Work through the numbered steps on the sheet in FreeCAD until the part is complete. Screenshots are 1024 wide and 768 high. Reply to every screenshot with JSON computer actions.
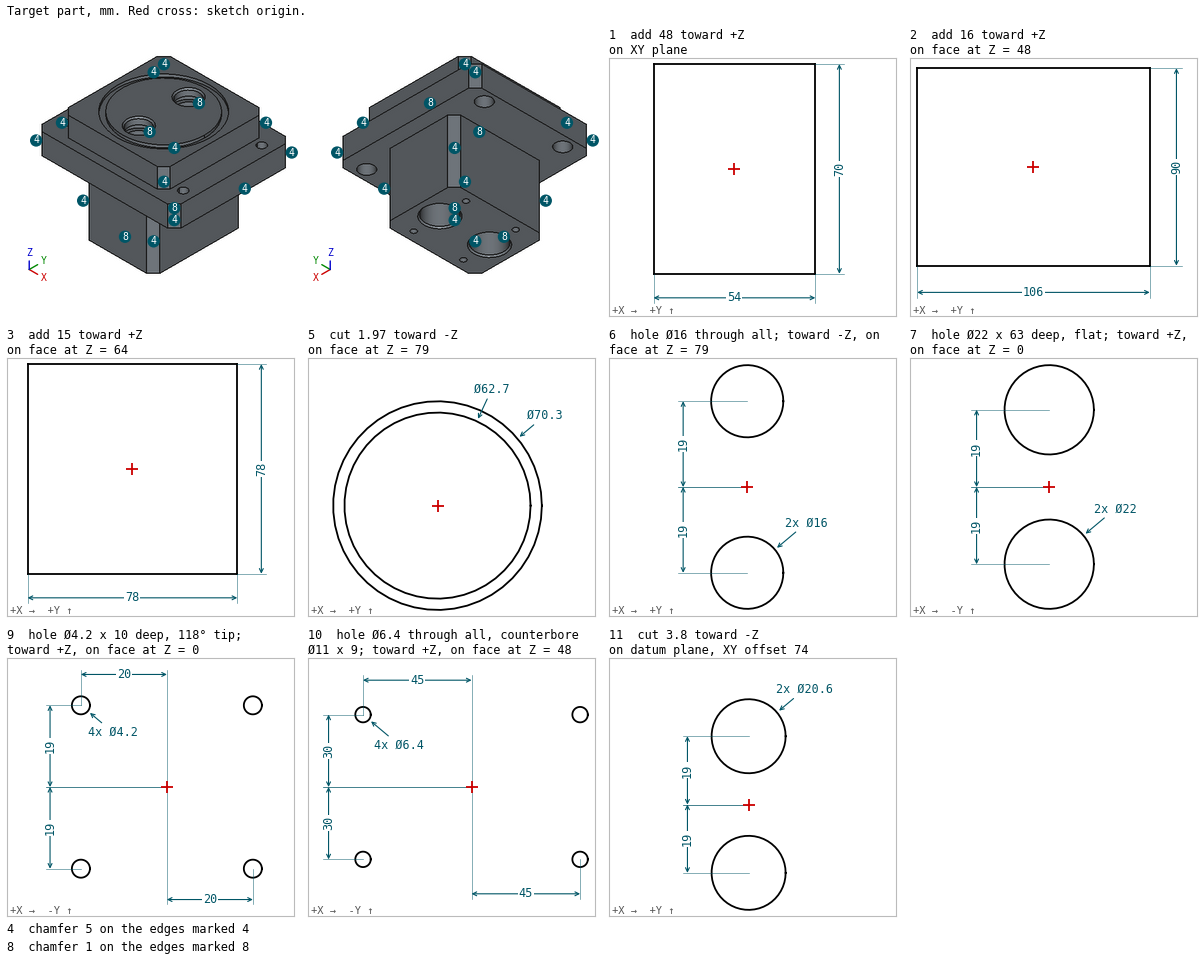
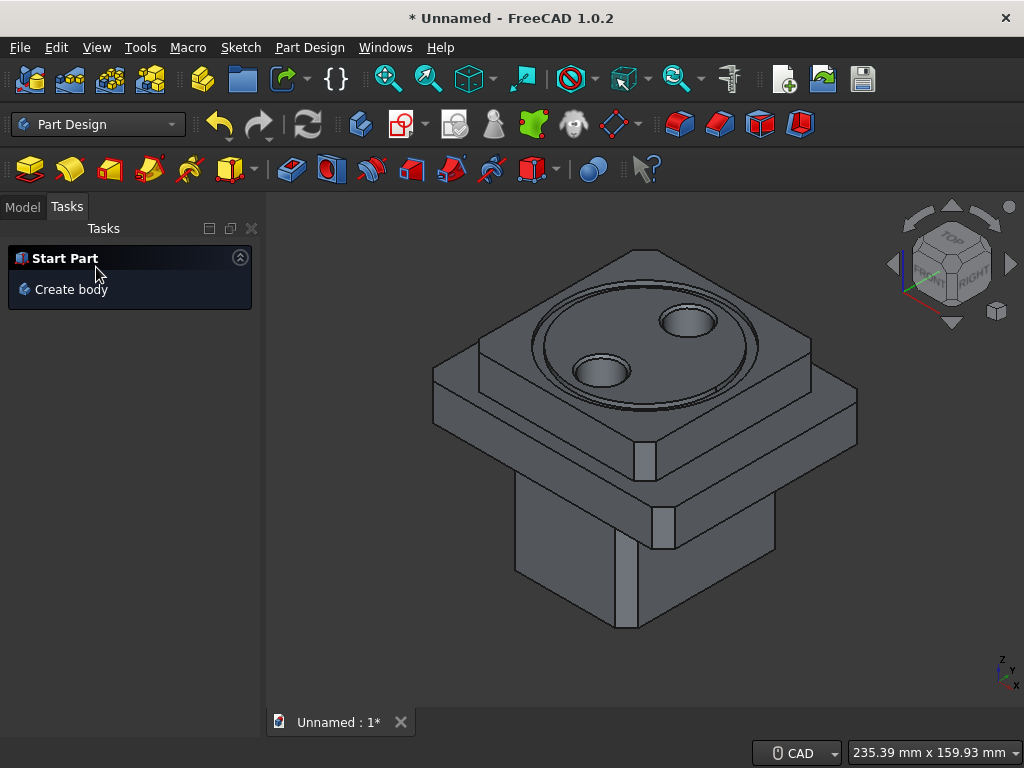
{"action": "key", "text": "5"}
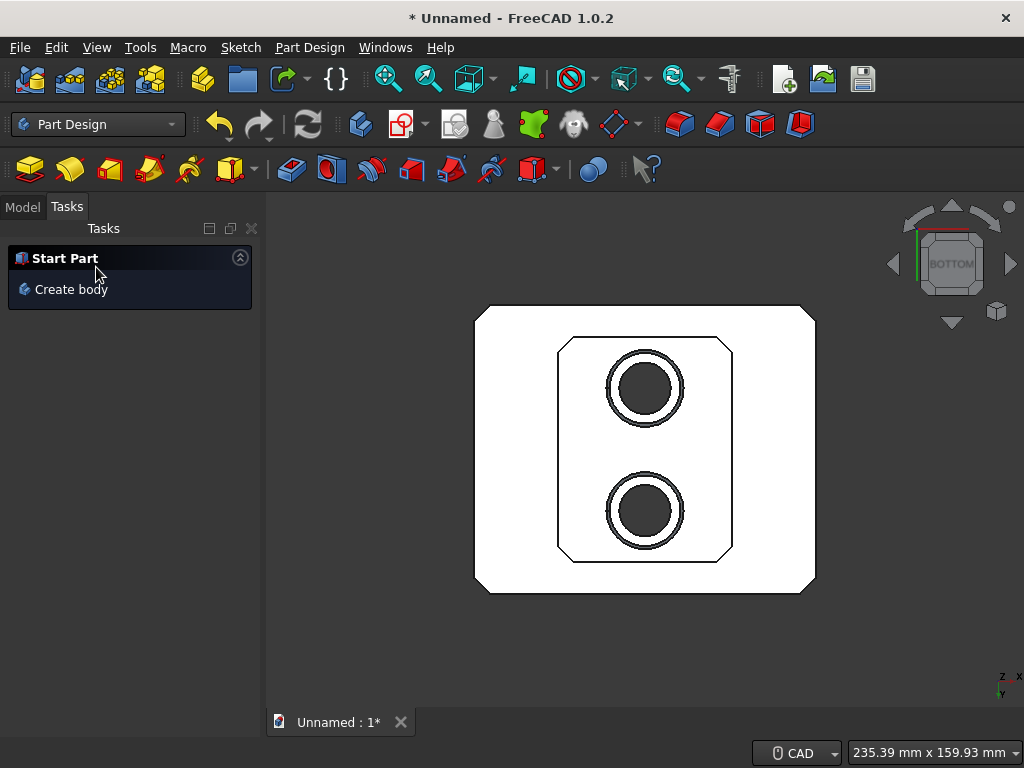
{"action": "left_click", "coordinate": [595, 449]}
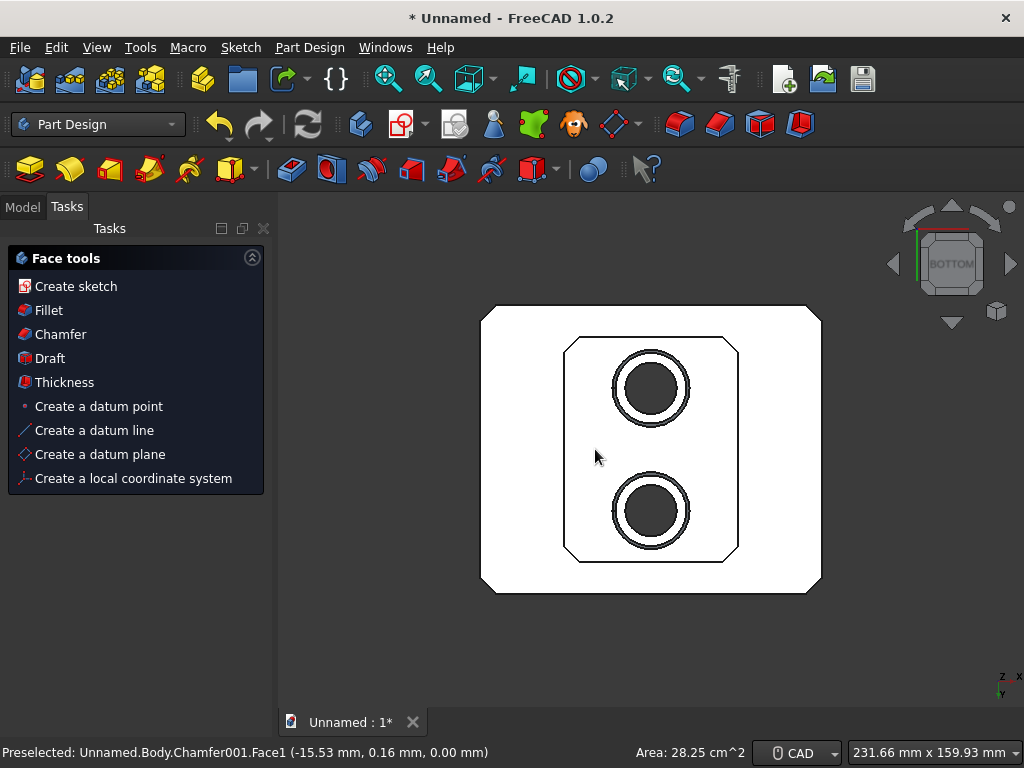
{"action": "left_click", "coordinate": [402, 124]}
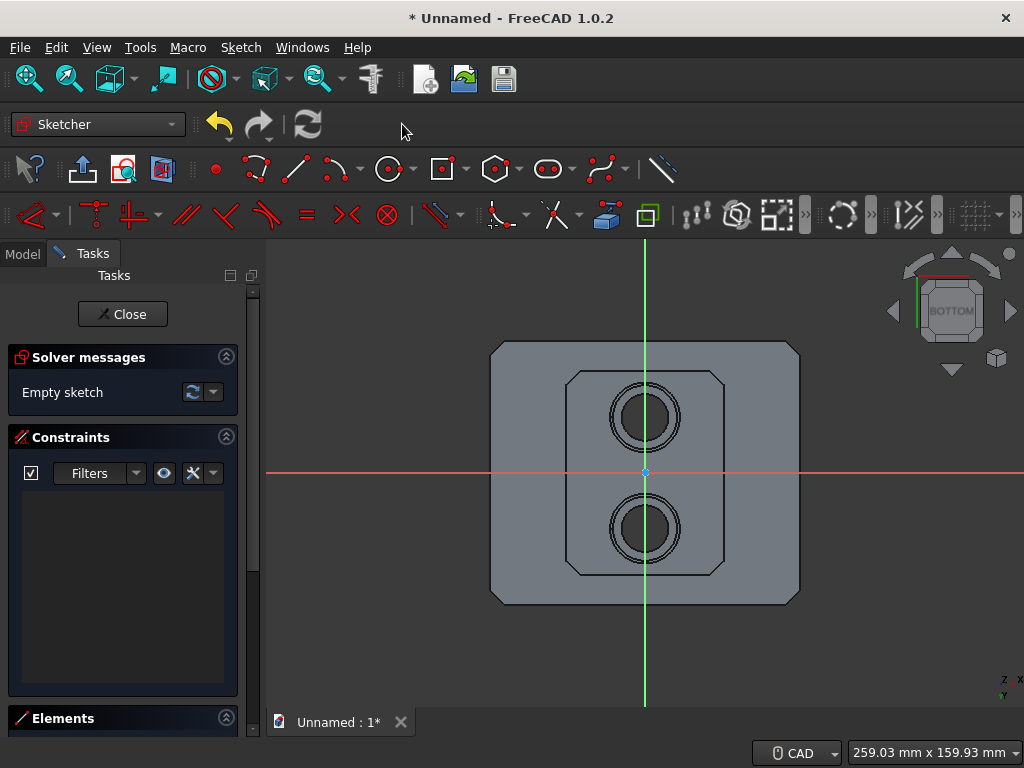
{"action": "scroll", "coordinate": [701, 473], "scroll_direction": "up", "scroll_amount": 4}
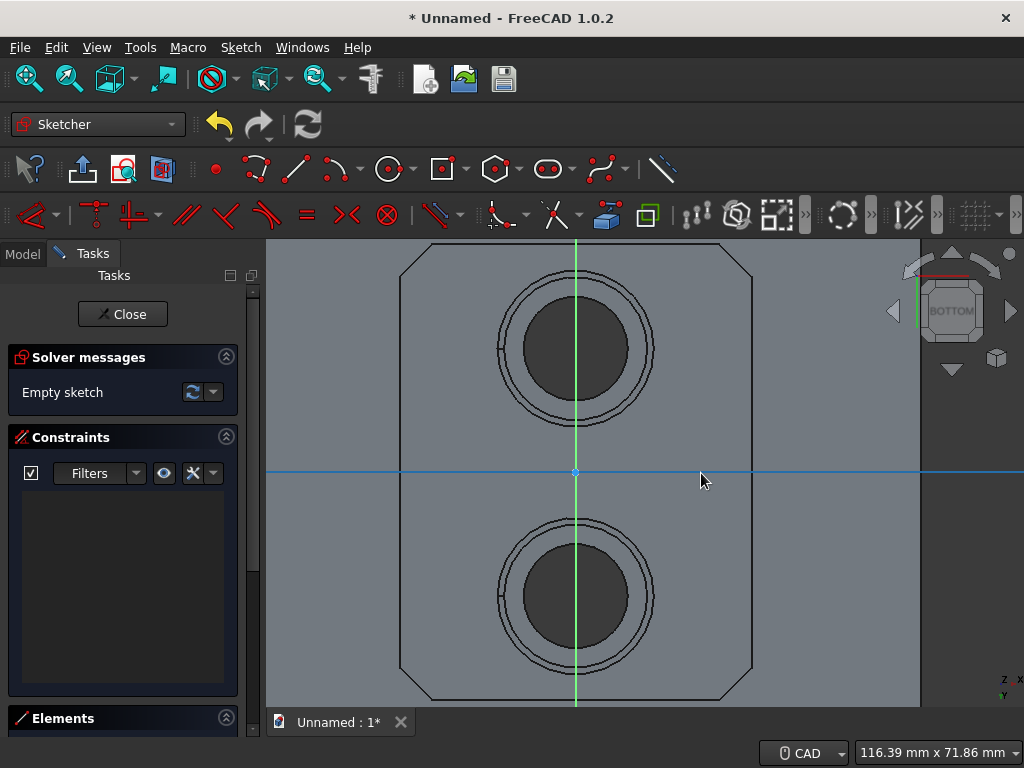
{"action": "left_click", "coordinate": [390, 170]}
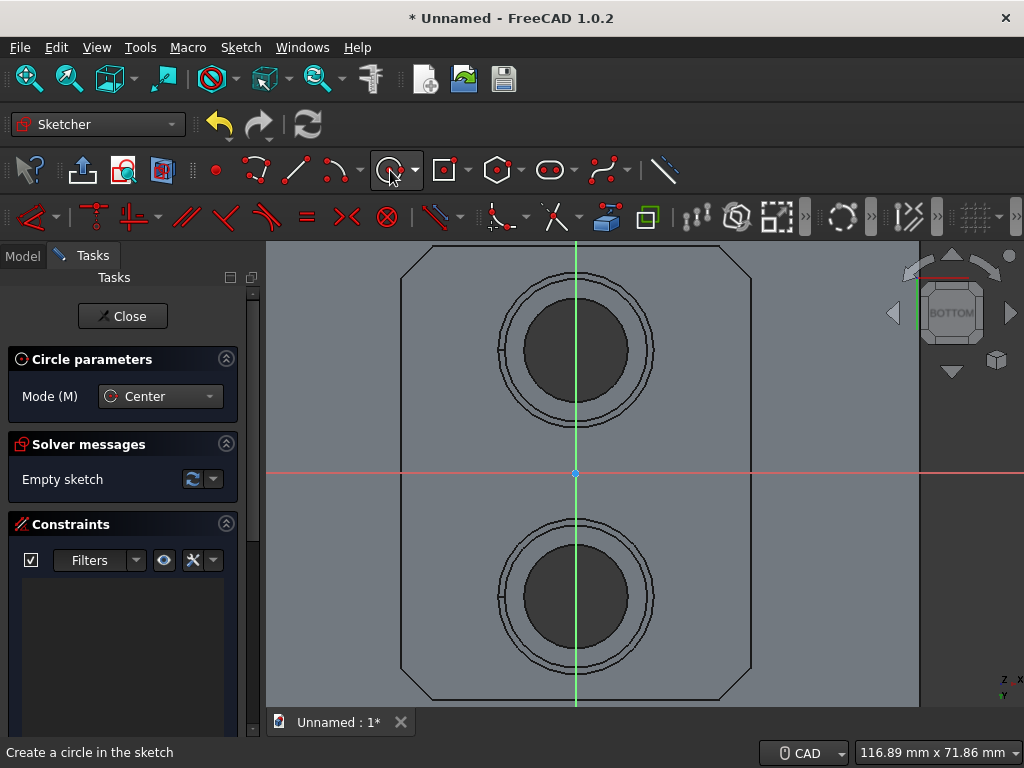
{"action": "scroll", "coordinate": [446, 350], "scroll_direction": "up", "scroll_amount": 3}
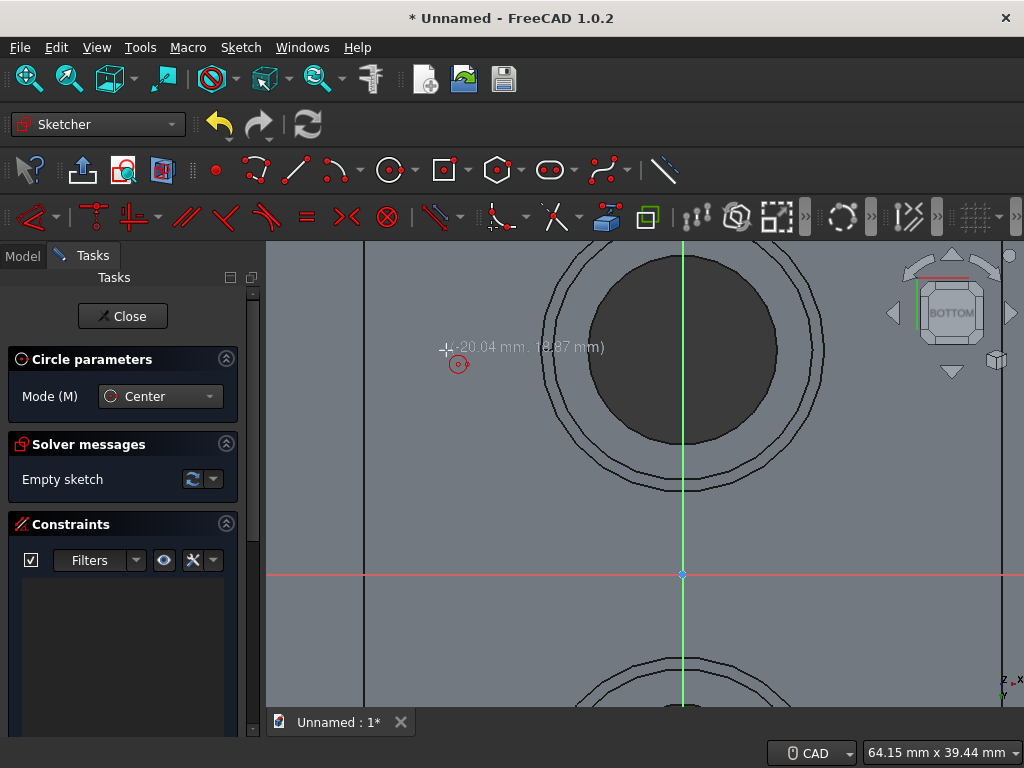
{"action": "left_click", "coordinate": [446, 350]}
{"action": "mouse_move", "coordinate": [464, 333]}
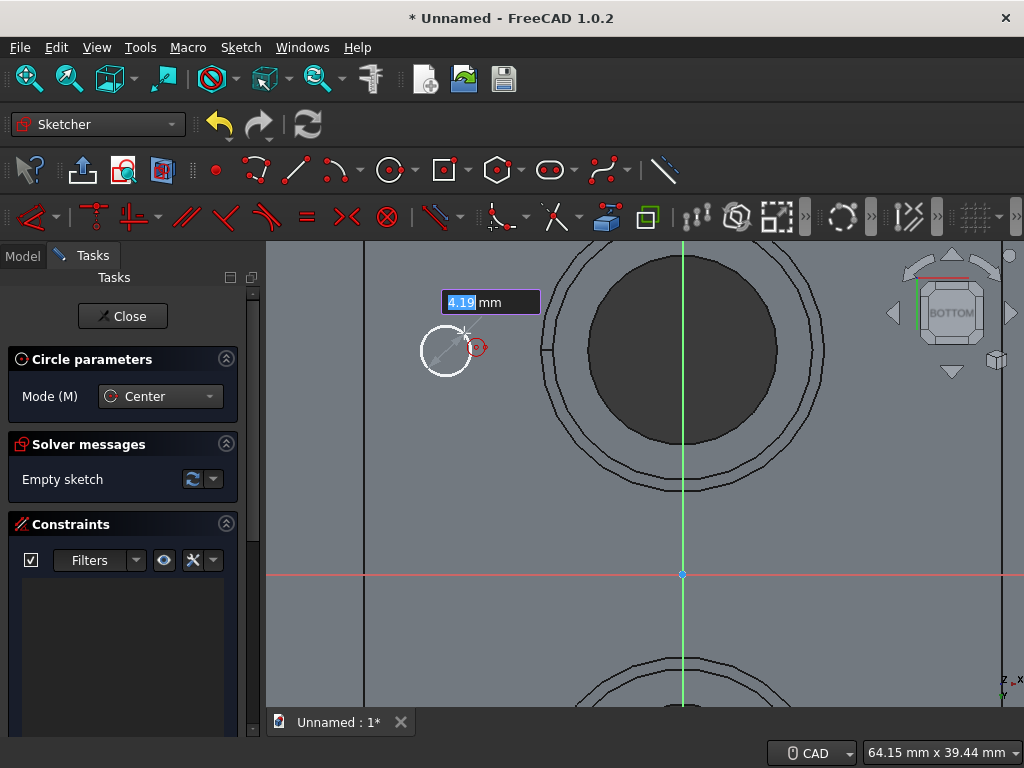
{"action": "type", "text": "4.2"}
{"action": "key", "text": "Return"}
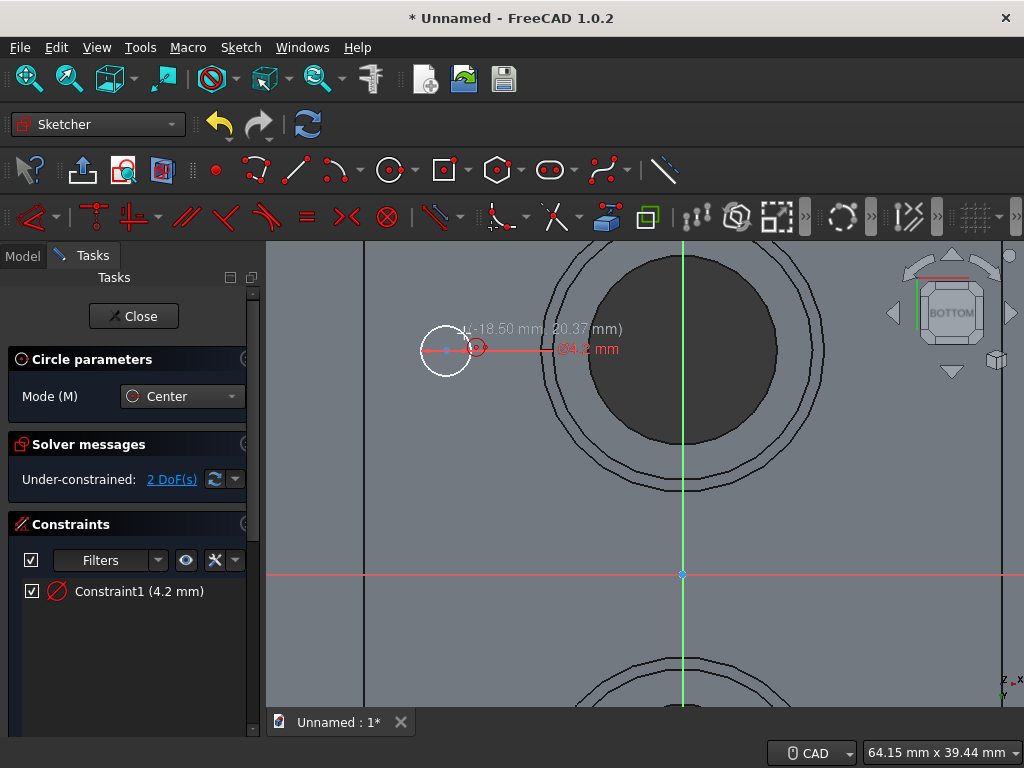
{"action": "scroll", "coordinate": [447, 352], "scroll_direction": "down", "scroll_amount": 3}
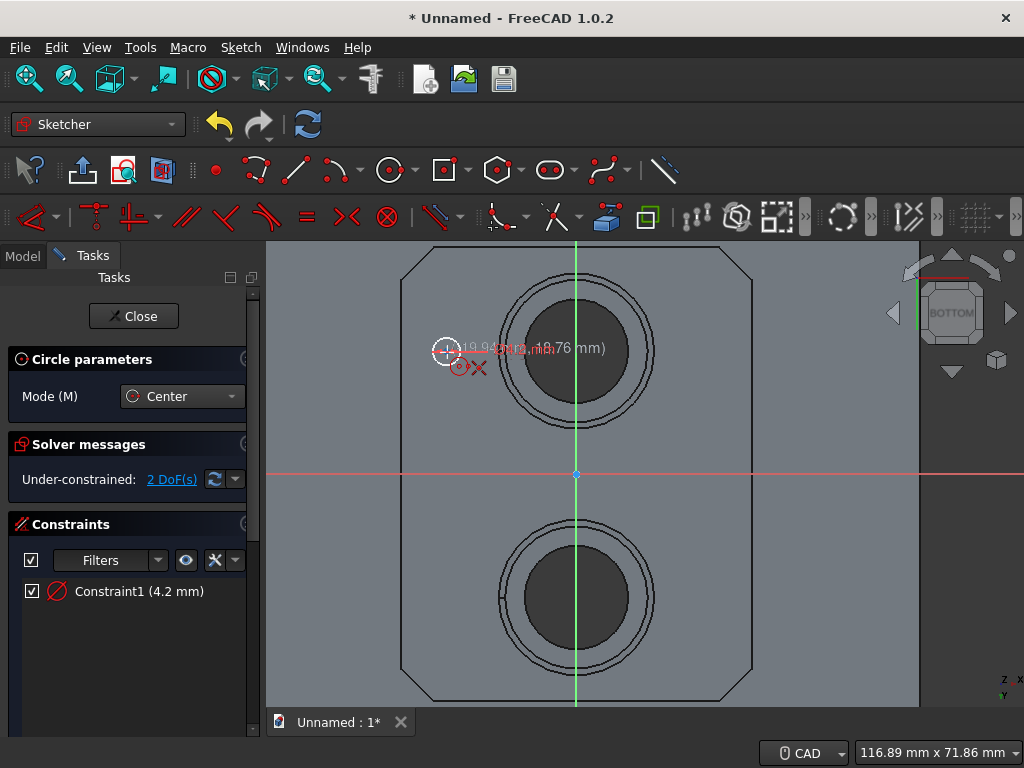
{"action": "scroll", "coordinate": [447, 598], "scroll_direction": "up", "scroll_amount": 3}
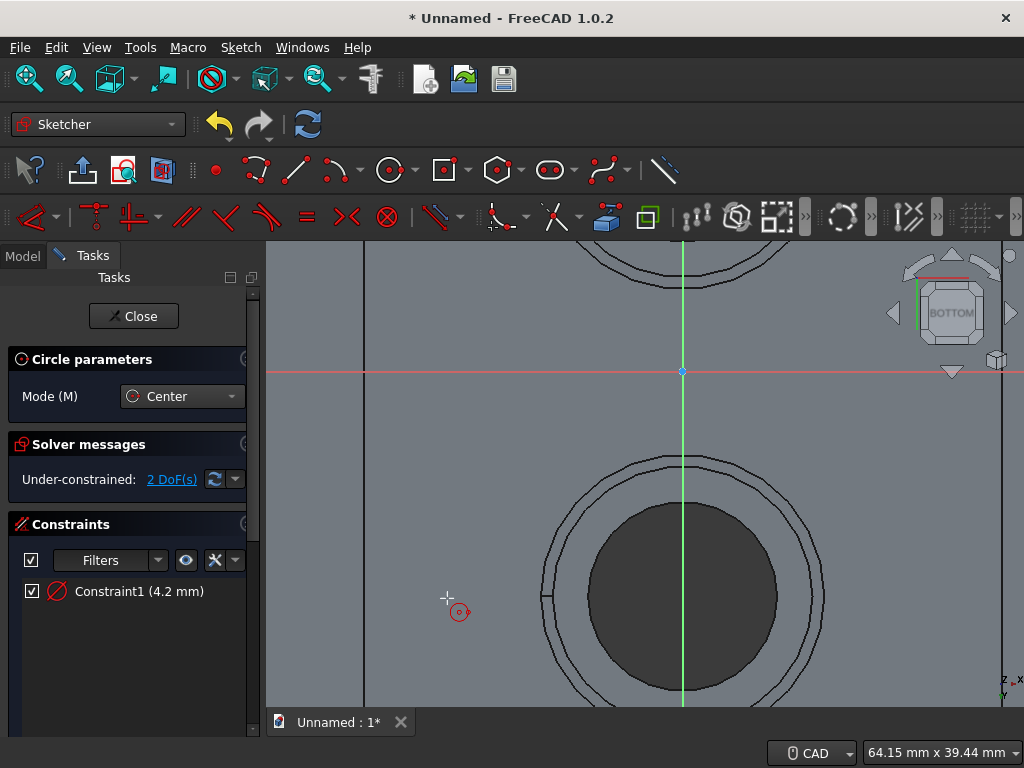
{"action": "left_click", "coordinate": [446, 596]}
{"action": "mouse_move", "coordinate": [464, 579]}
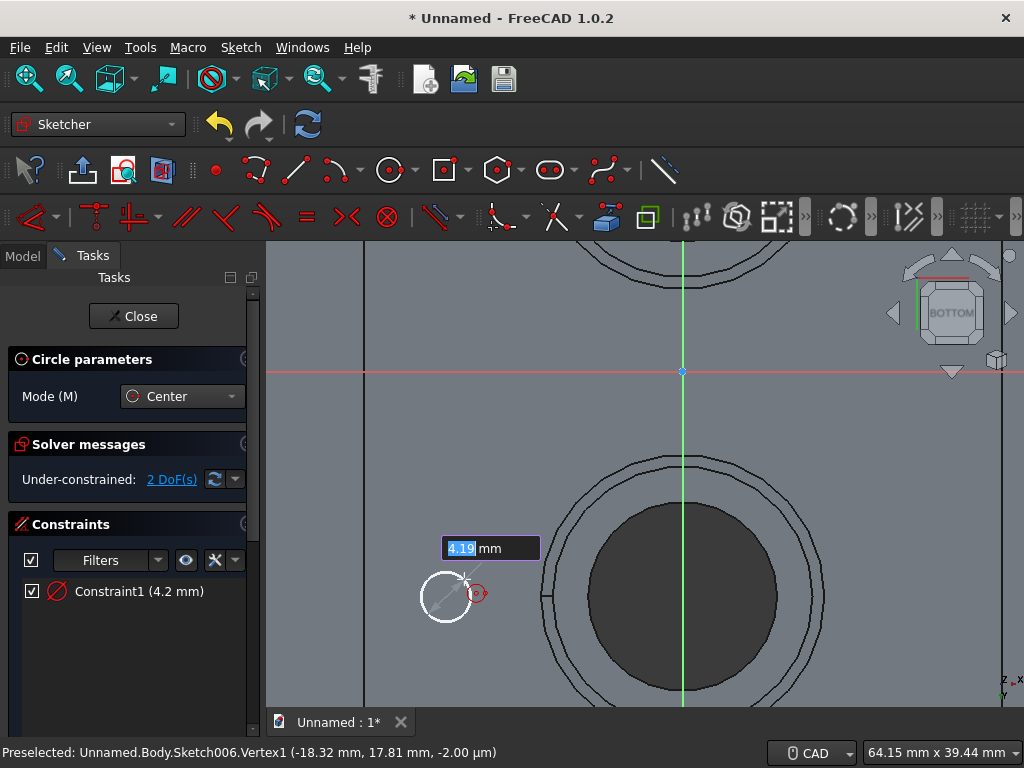
{"action": "type", "text": "4.2"}
{"action": "key", "text": "Return"}